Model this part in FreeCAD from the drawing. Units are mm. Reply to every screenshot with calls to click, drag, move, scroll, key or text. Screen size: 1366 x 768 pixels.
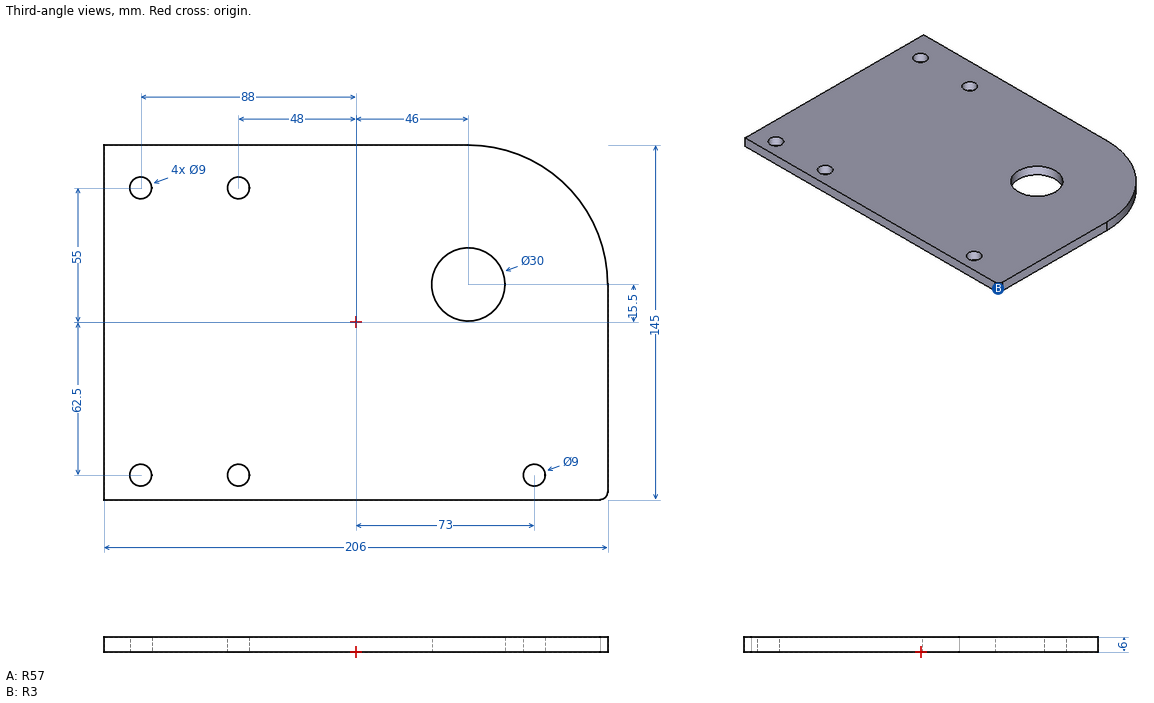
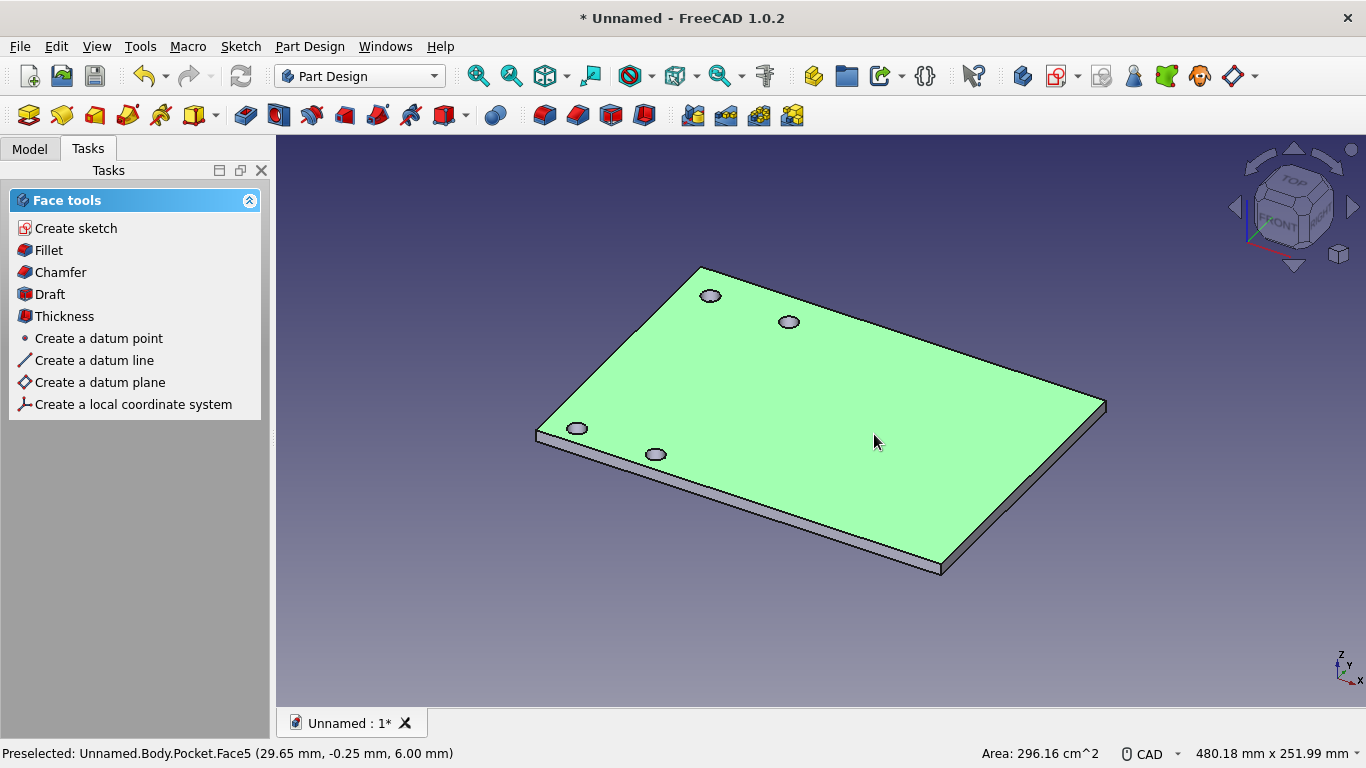
click(1056, 76)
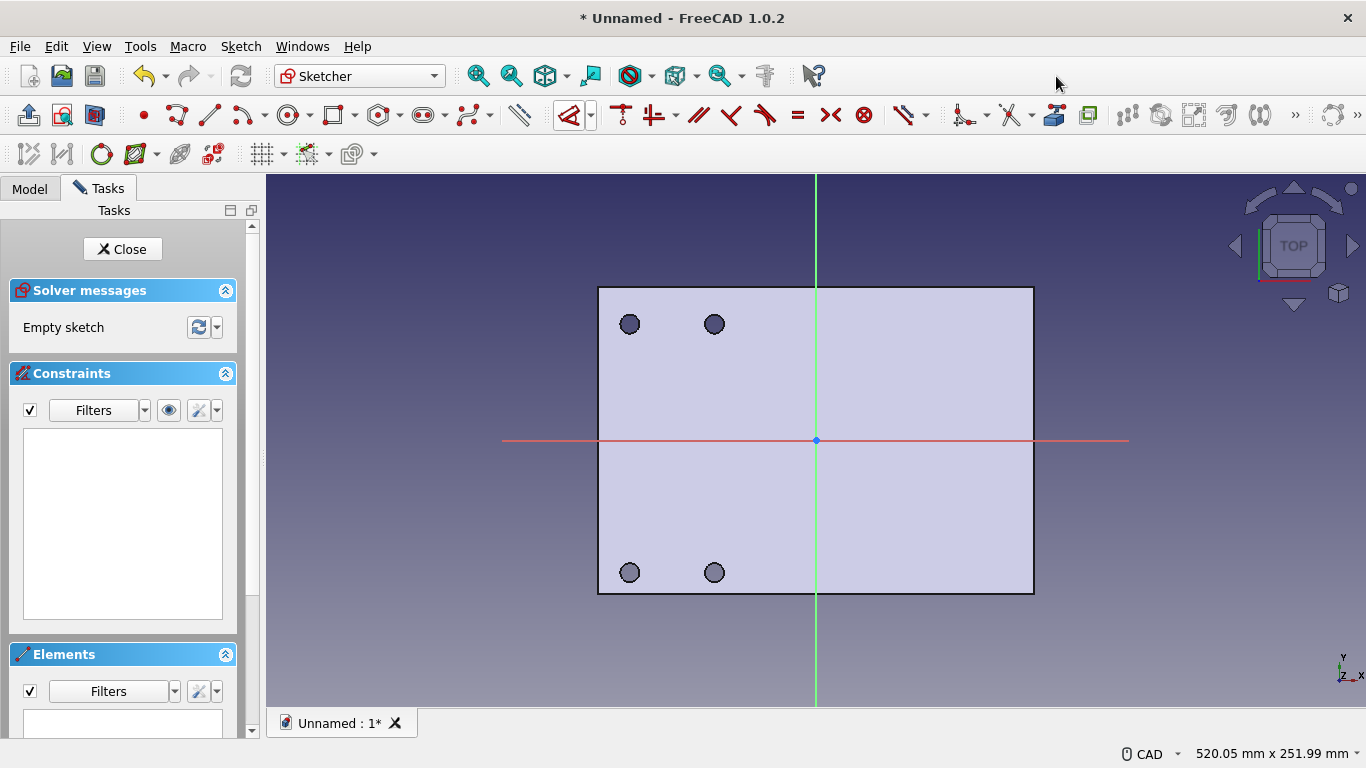
scroll(914, 400, up, 8)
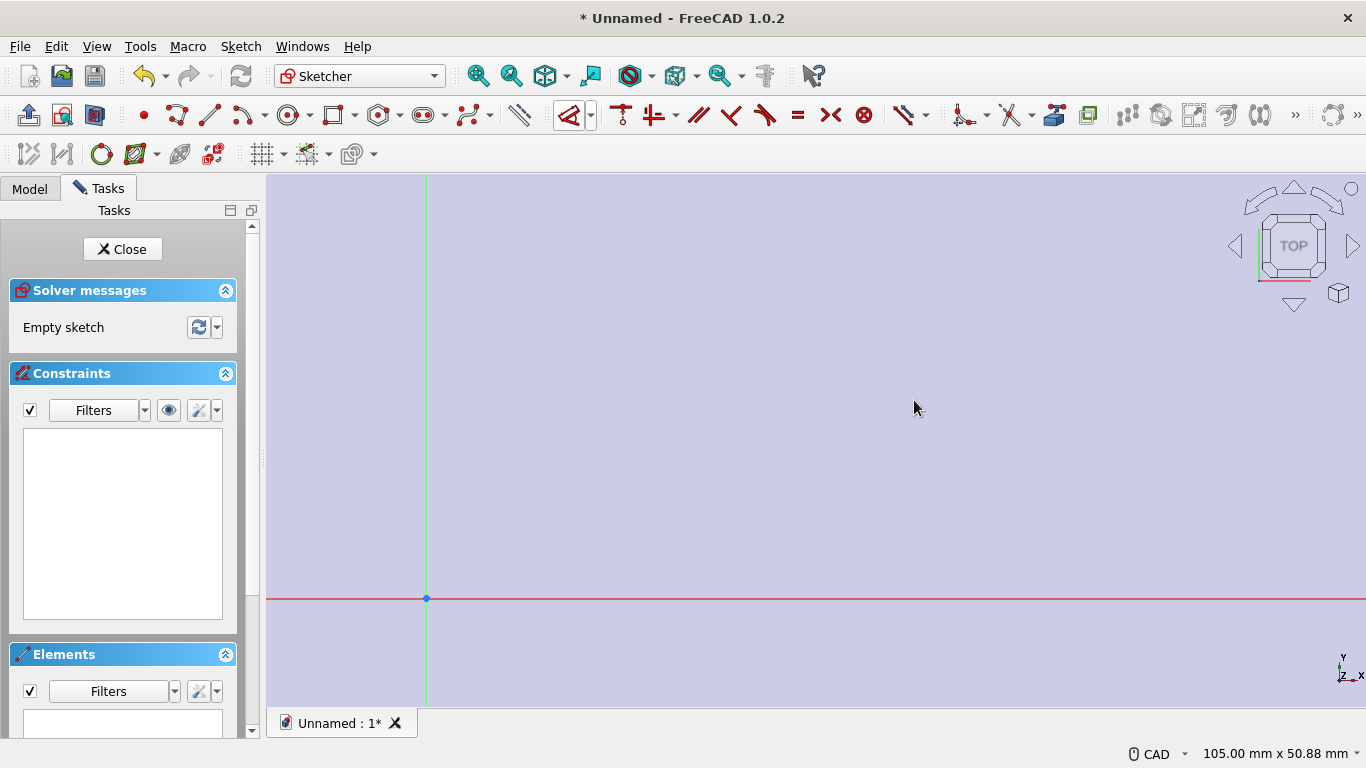
click(288, 116)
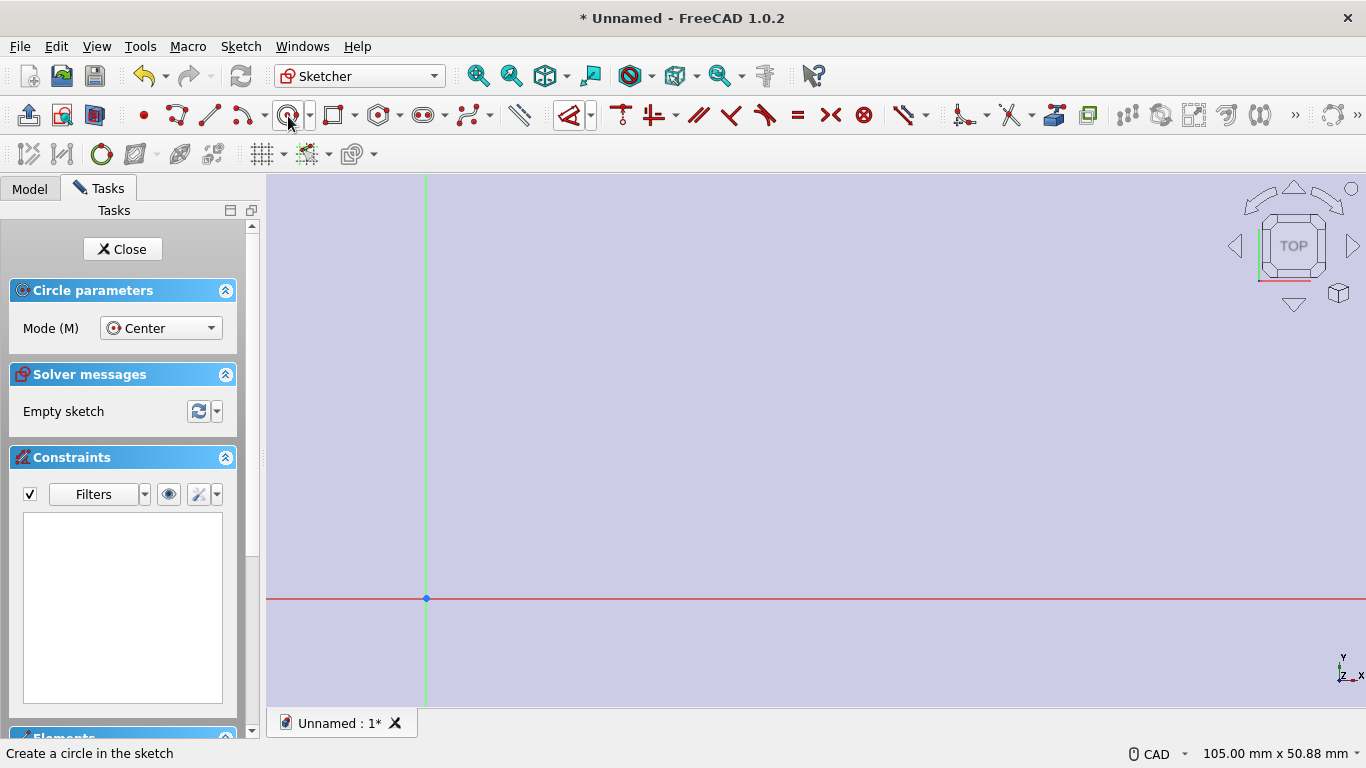
click(908, 437)
move(1019, 325)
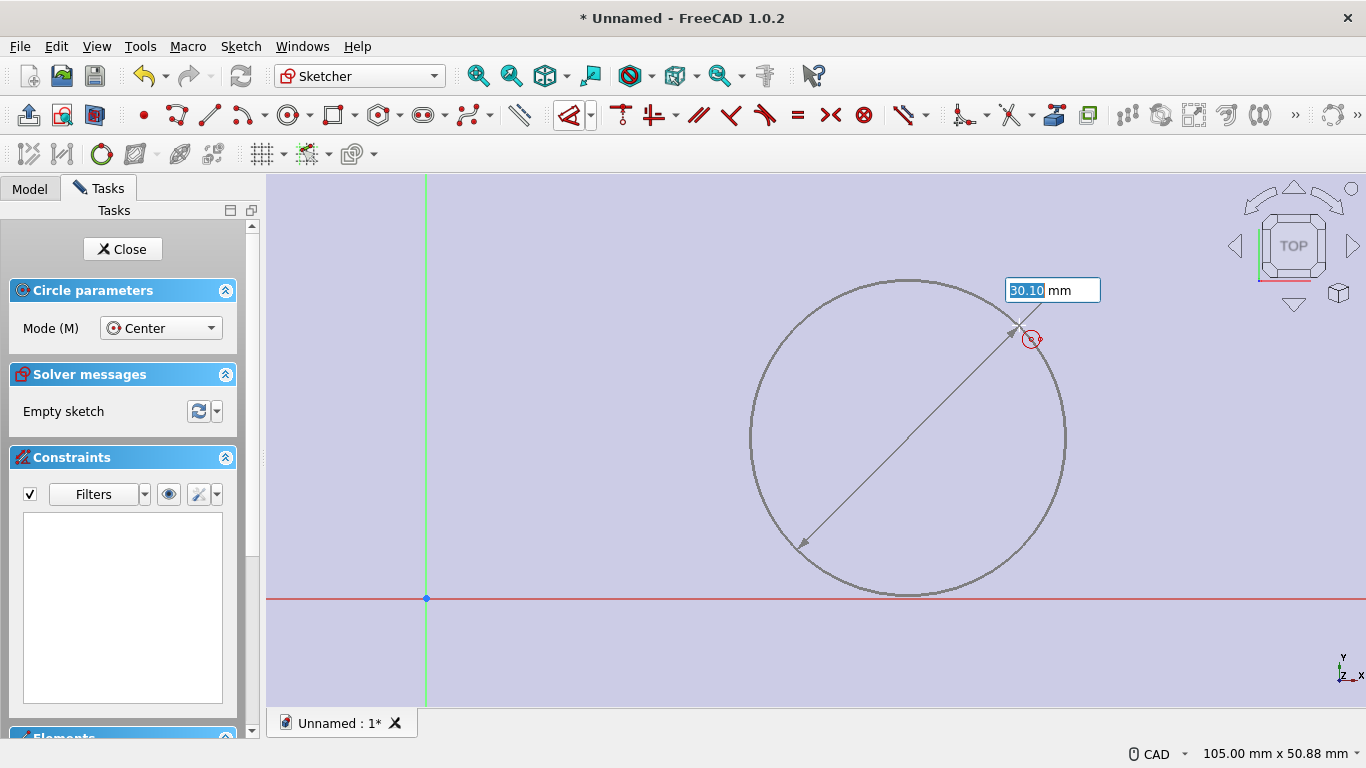
text(30)
key(Return)
key(Escape)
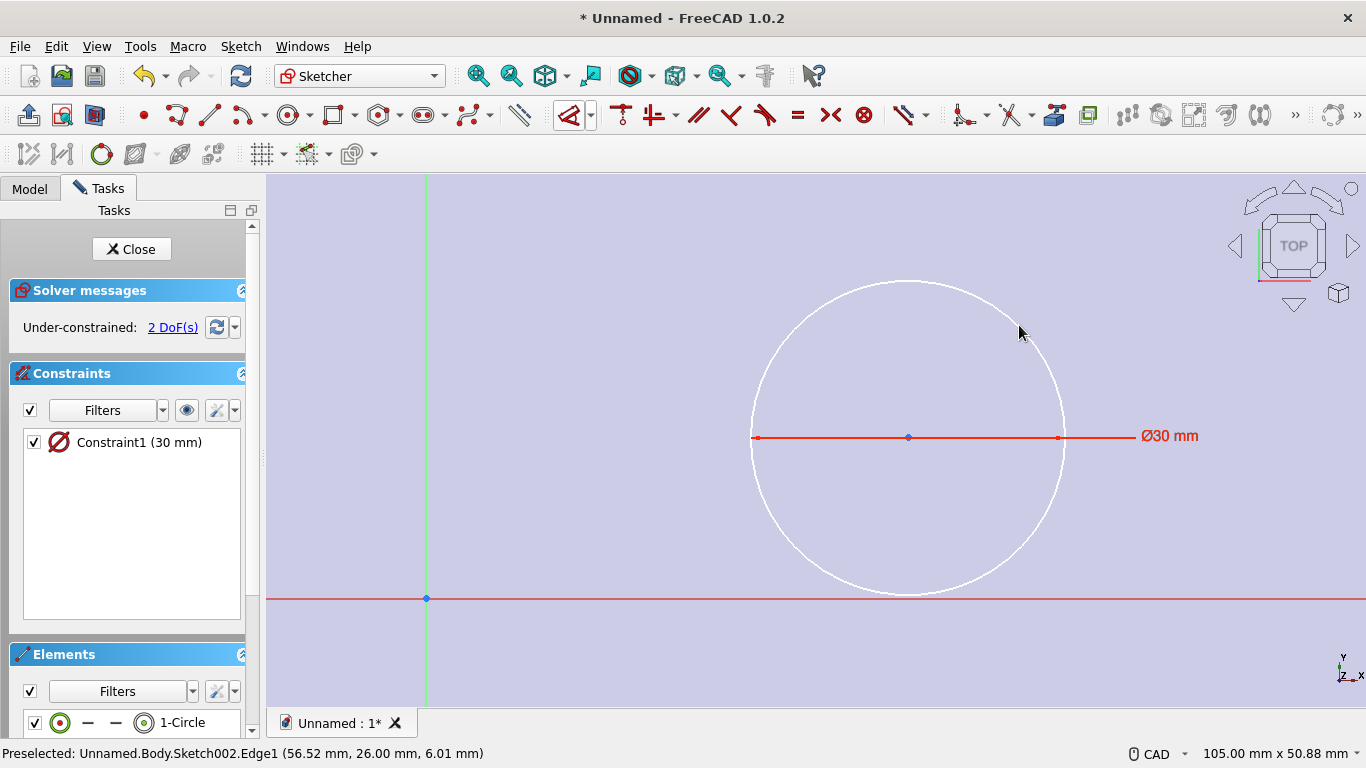
click(908, 438)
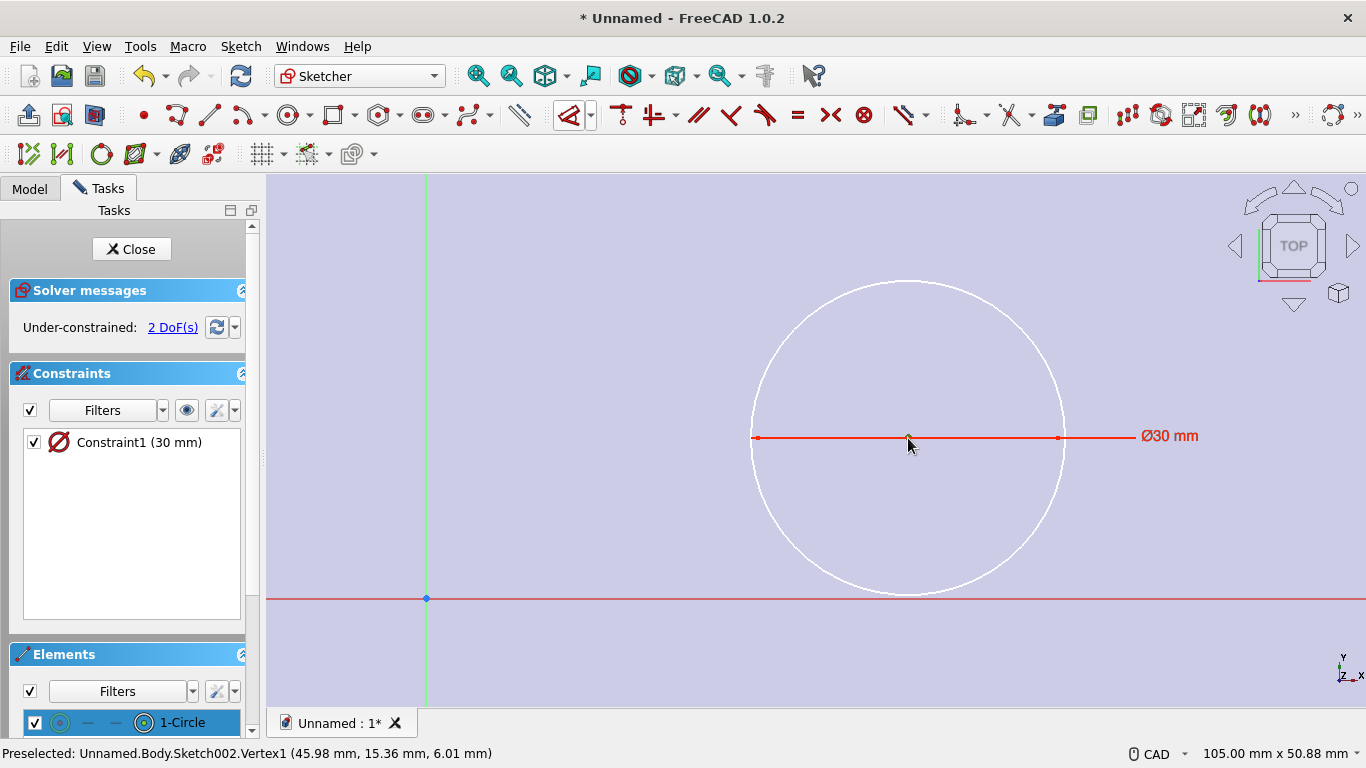
key(l)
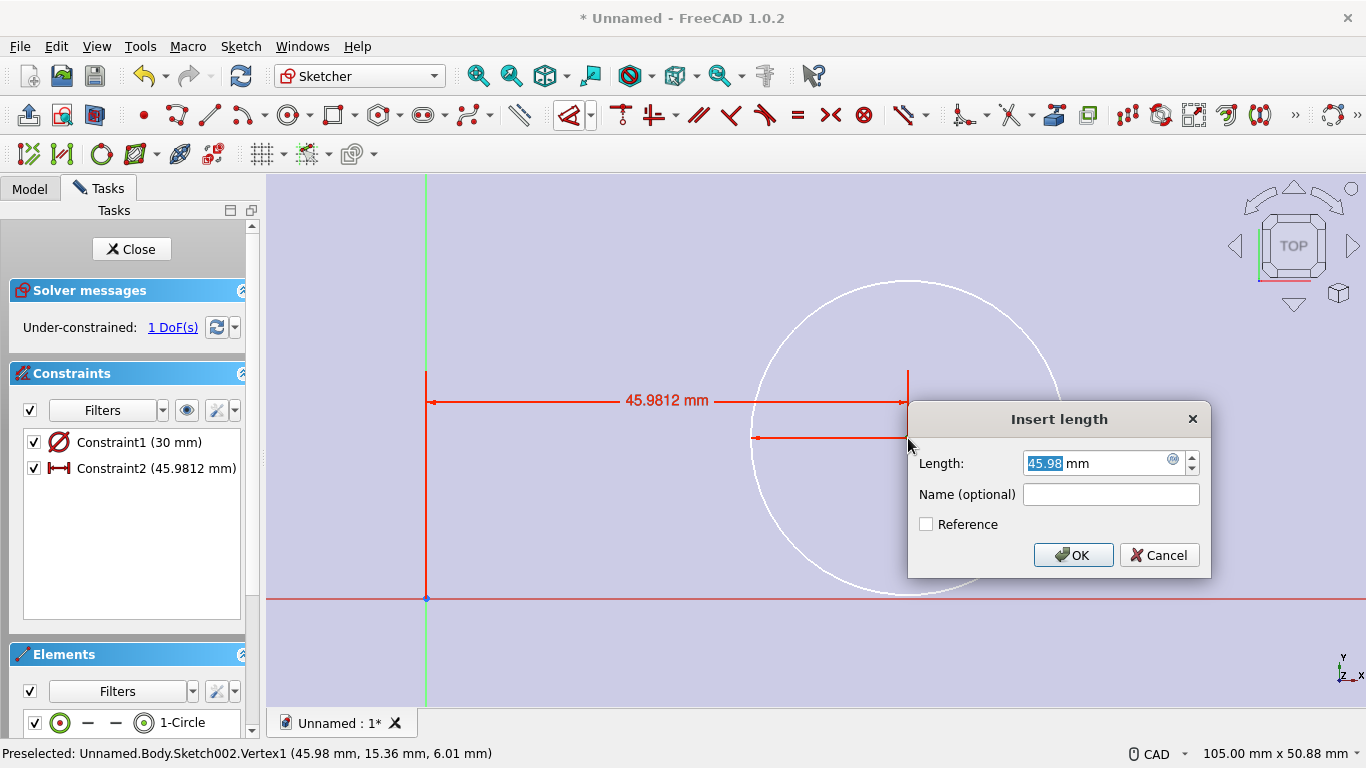
text(46)
key(Return)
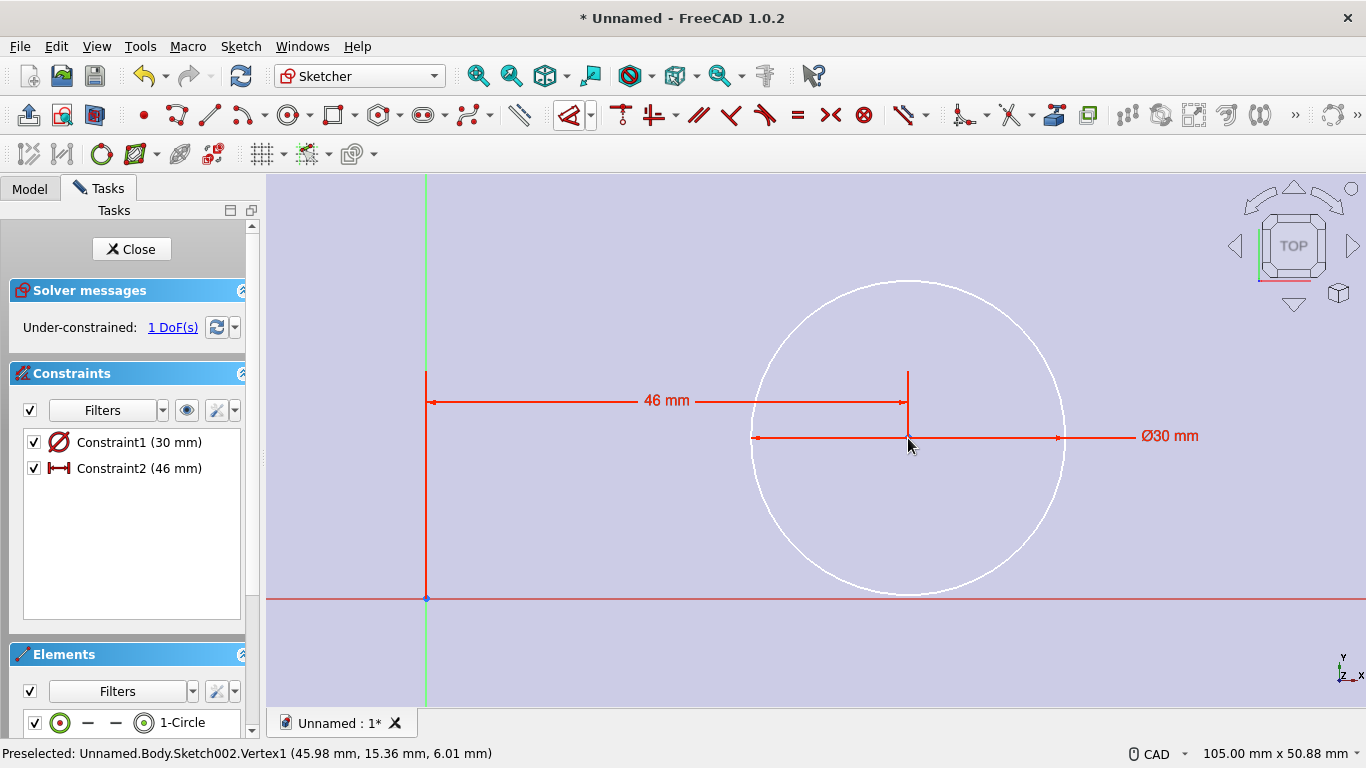
click(908, 438)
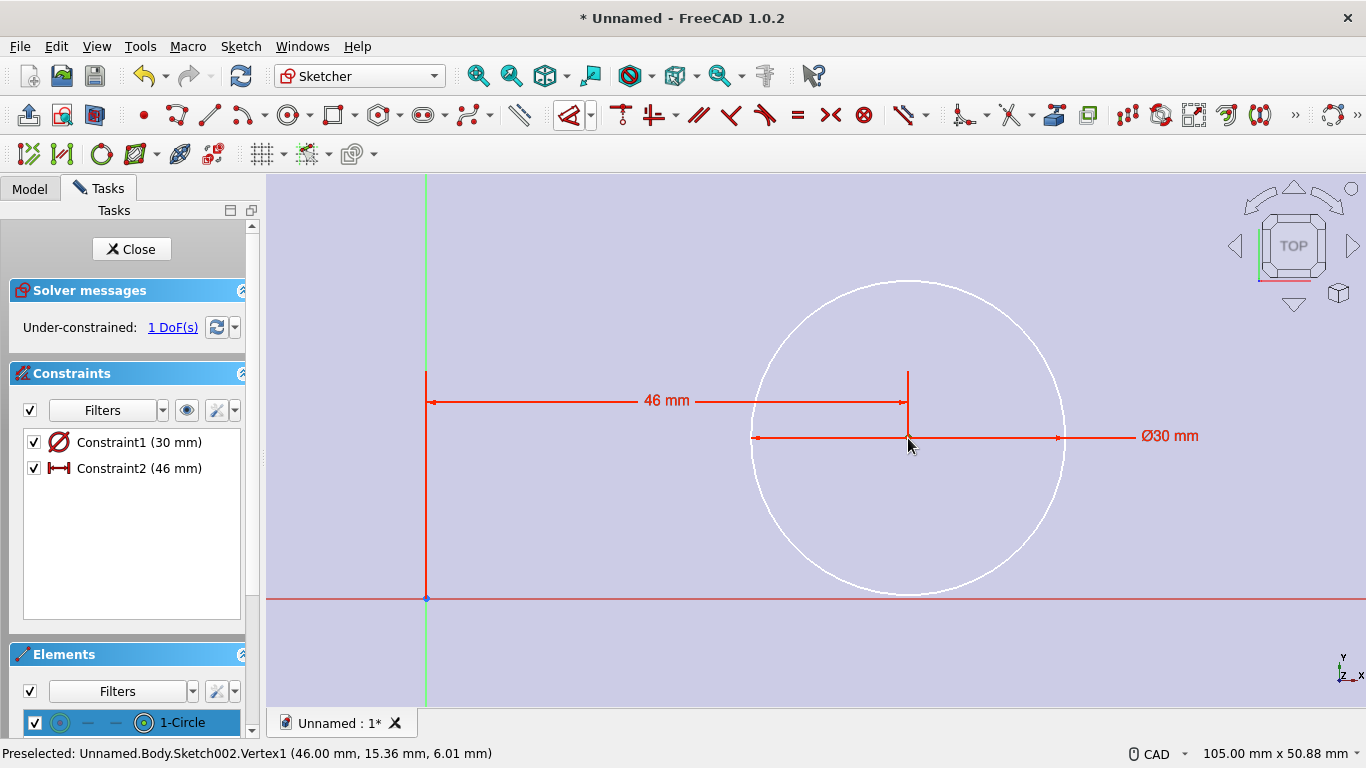
key(i)